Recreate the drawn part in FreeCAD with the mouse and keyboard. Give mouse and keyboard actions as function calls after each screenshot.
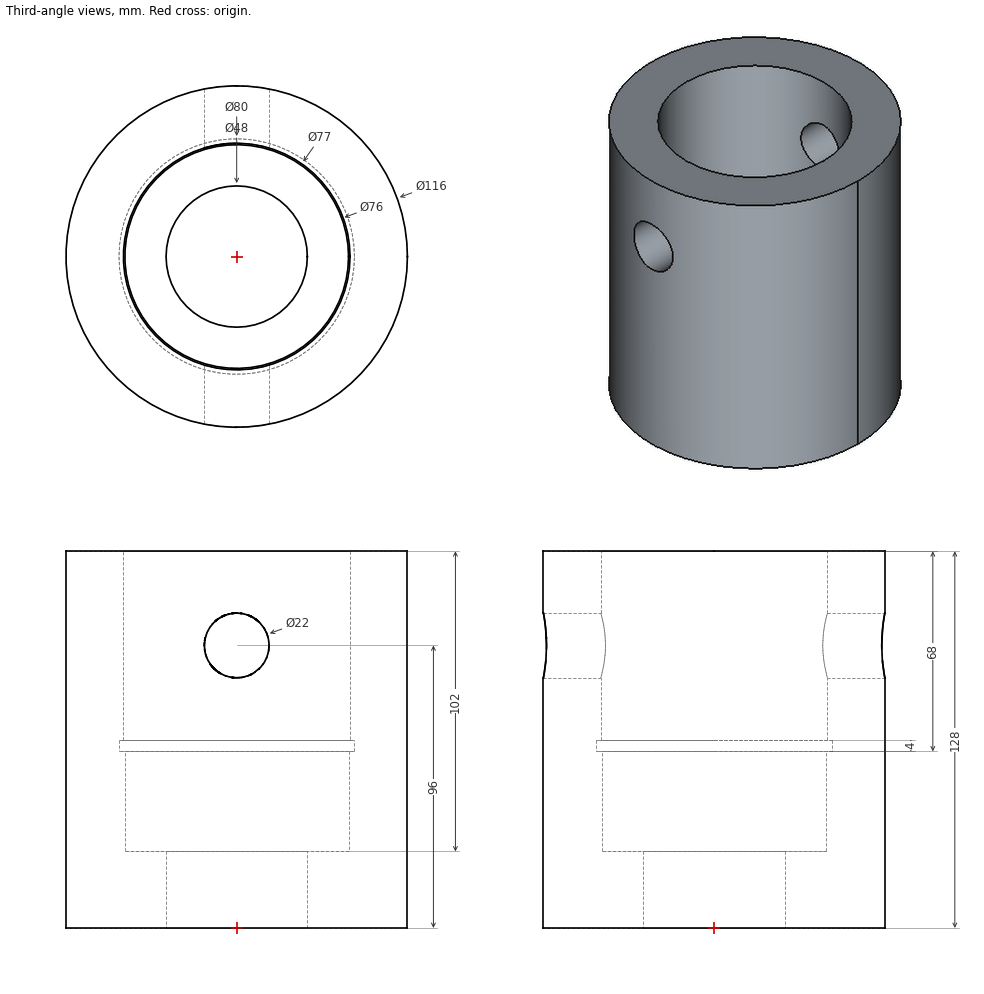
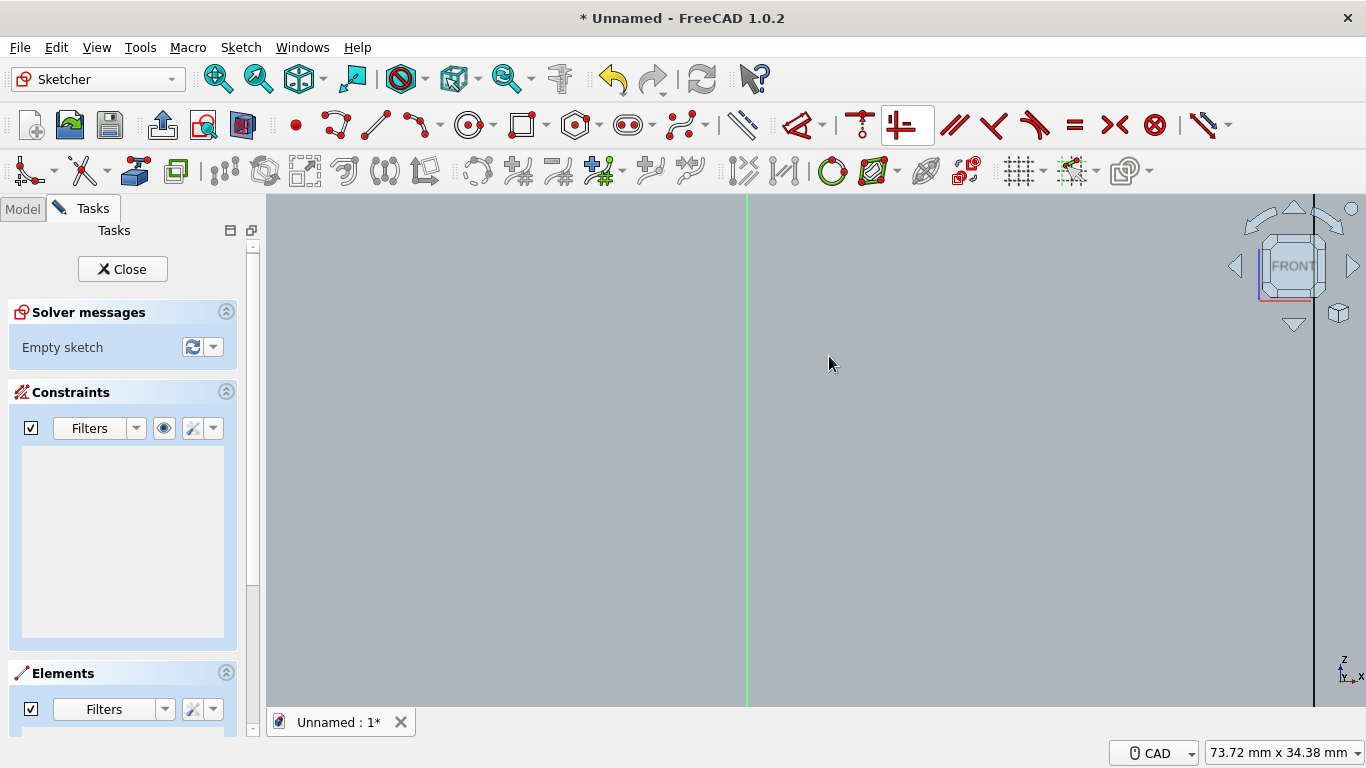
key(g)
key(c)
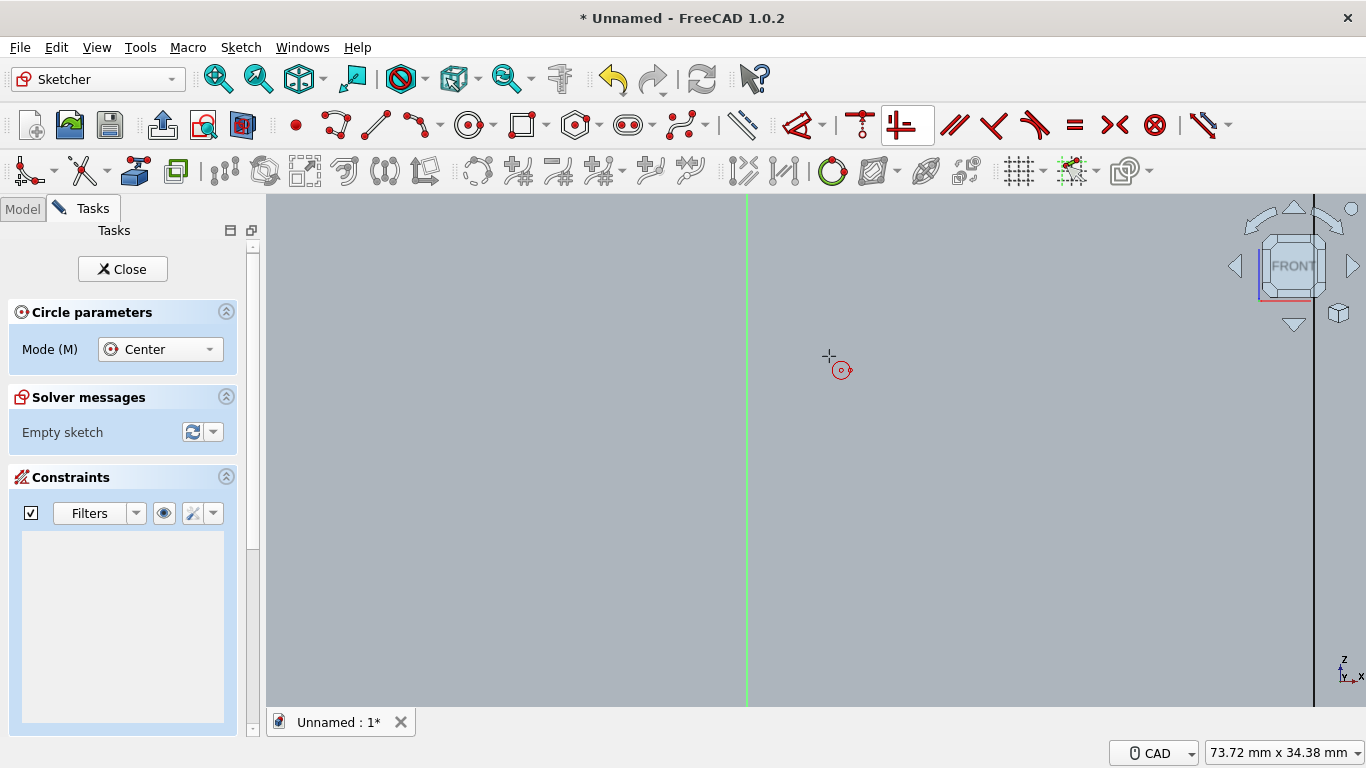
click(747, 449)
move(863, 333)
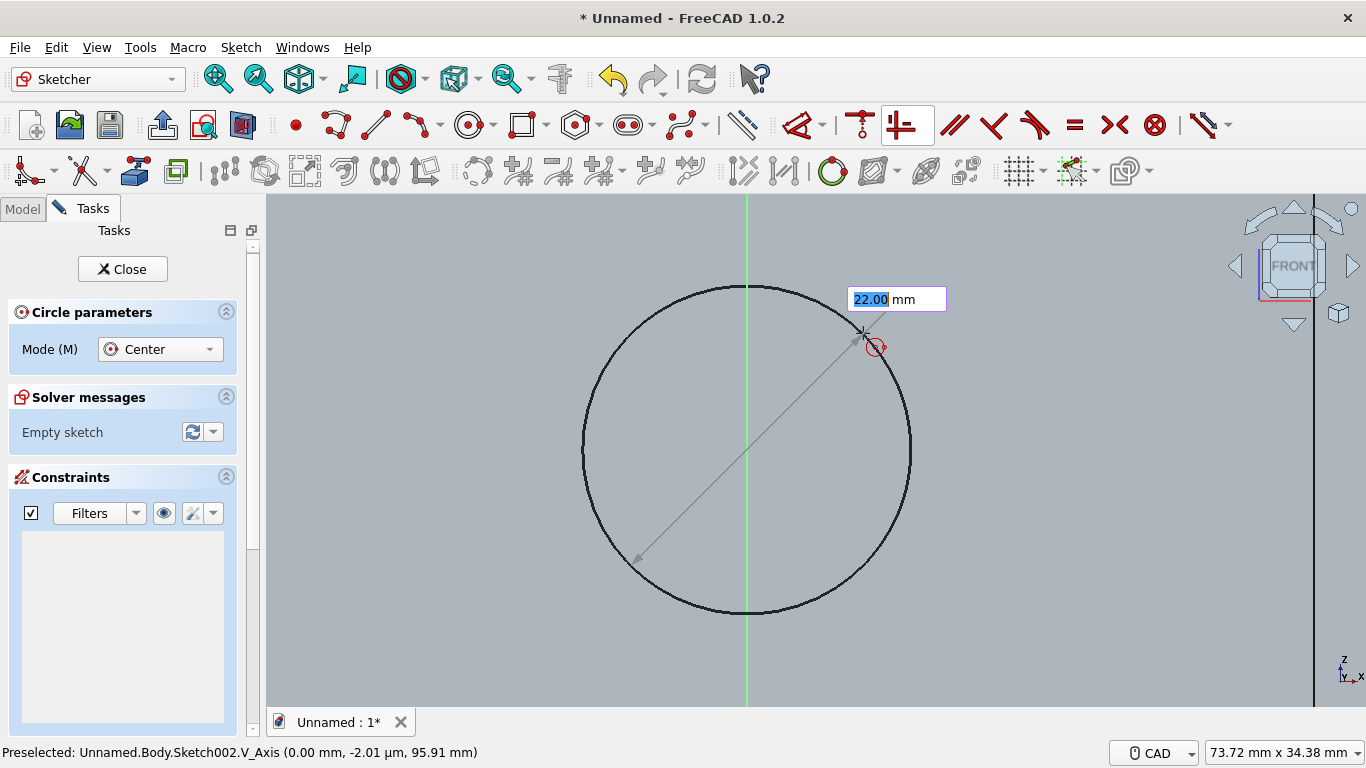
text(22)
key(Return)
key(Escape)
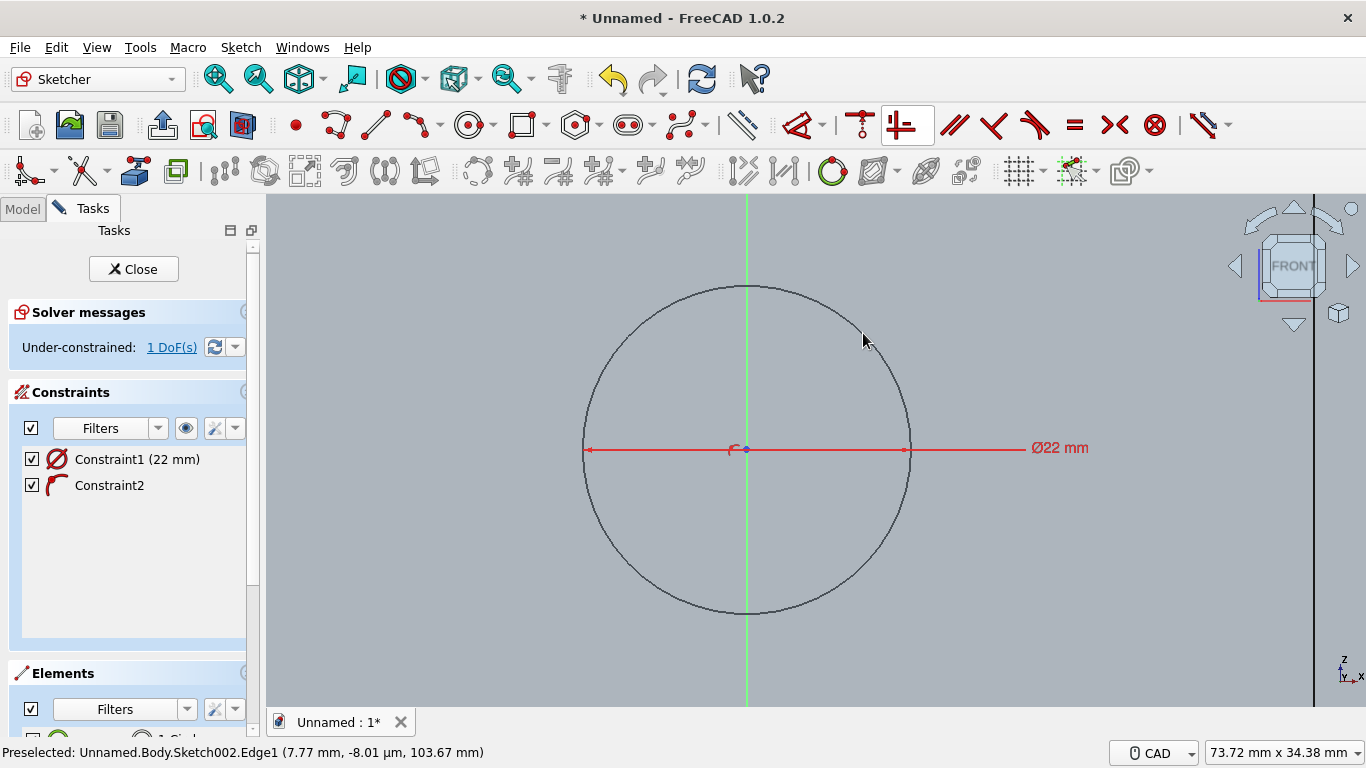
key(d)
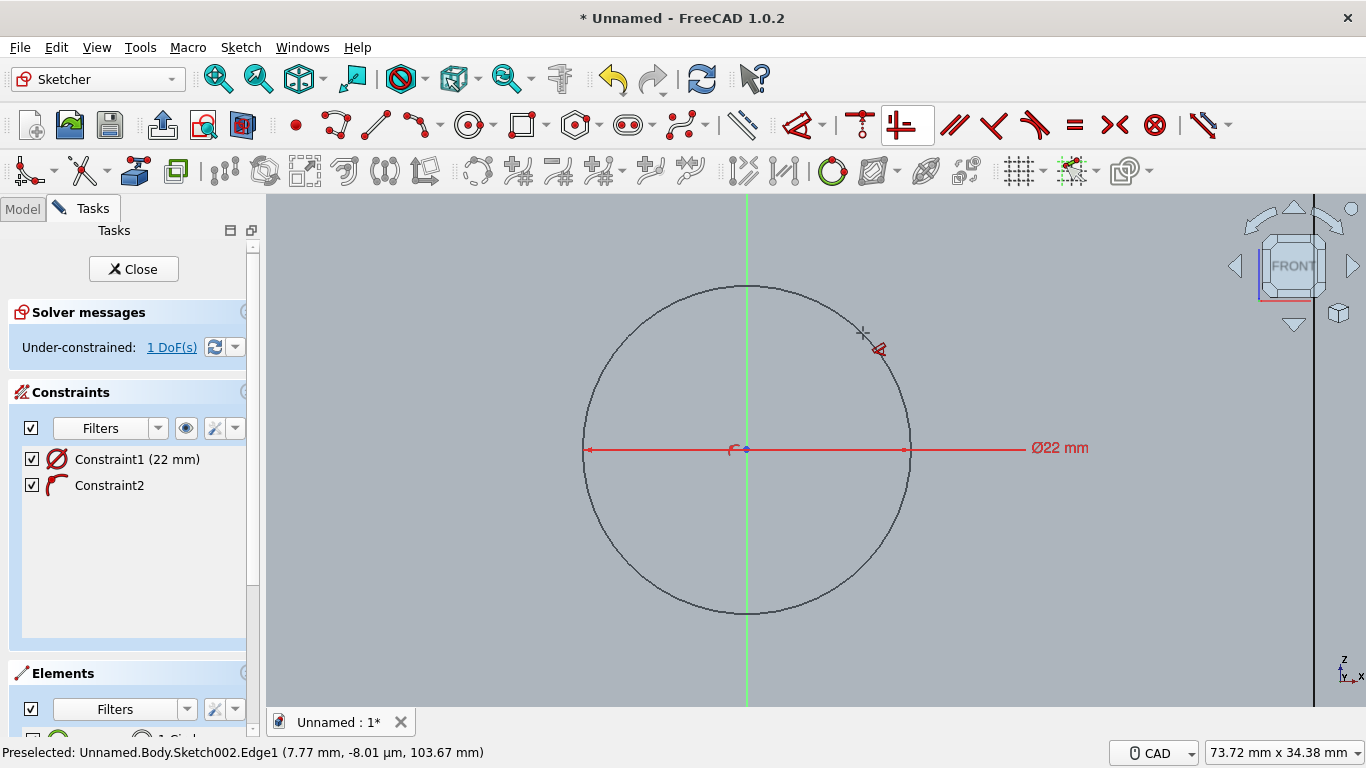
click(747, 450)
click(781, 564)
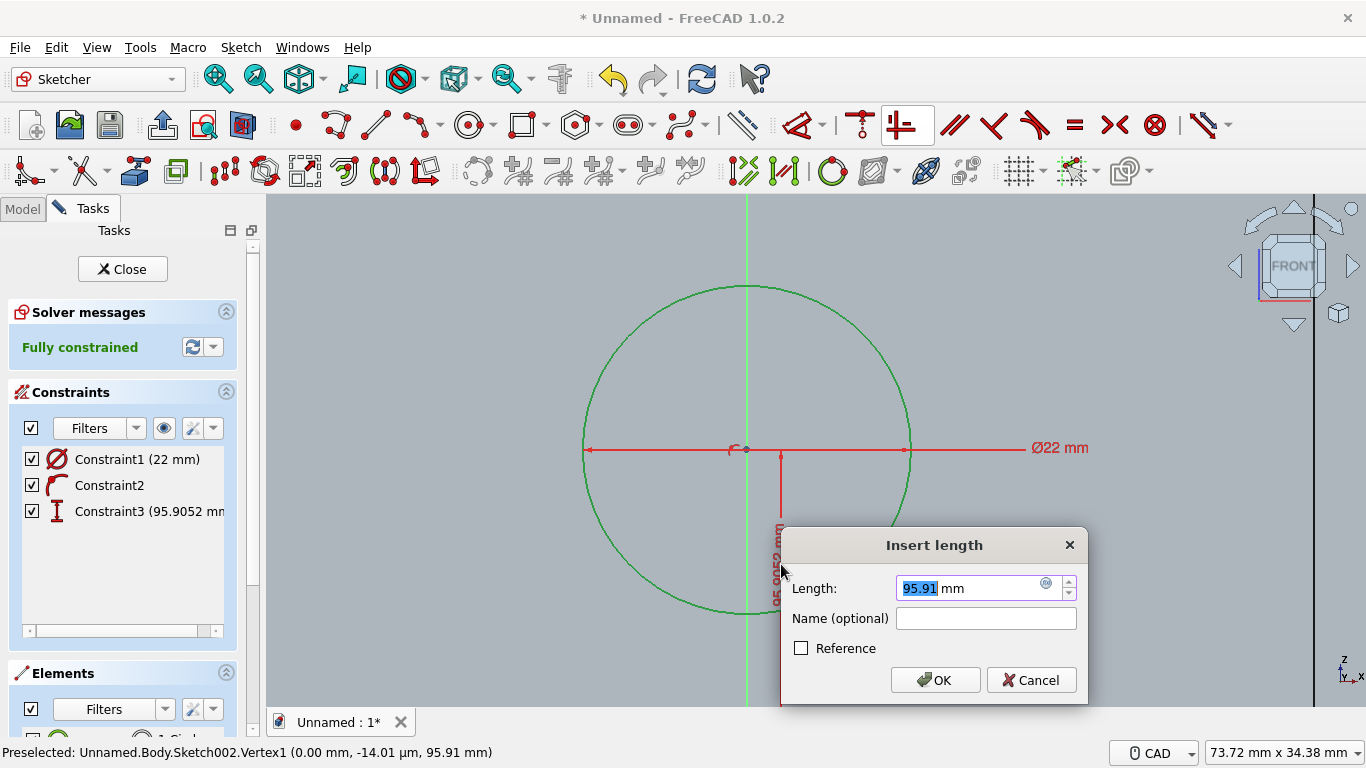
text(96)
key(Return)
key(Escape)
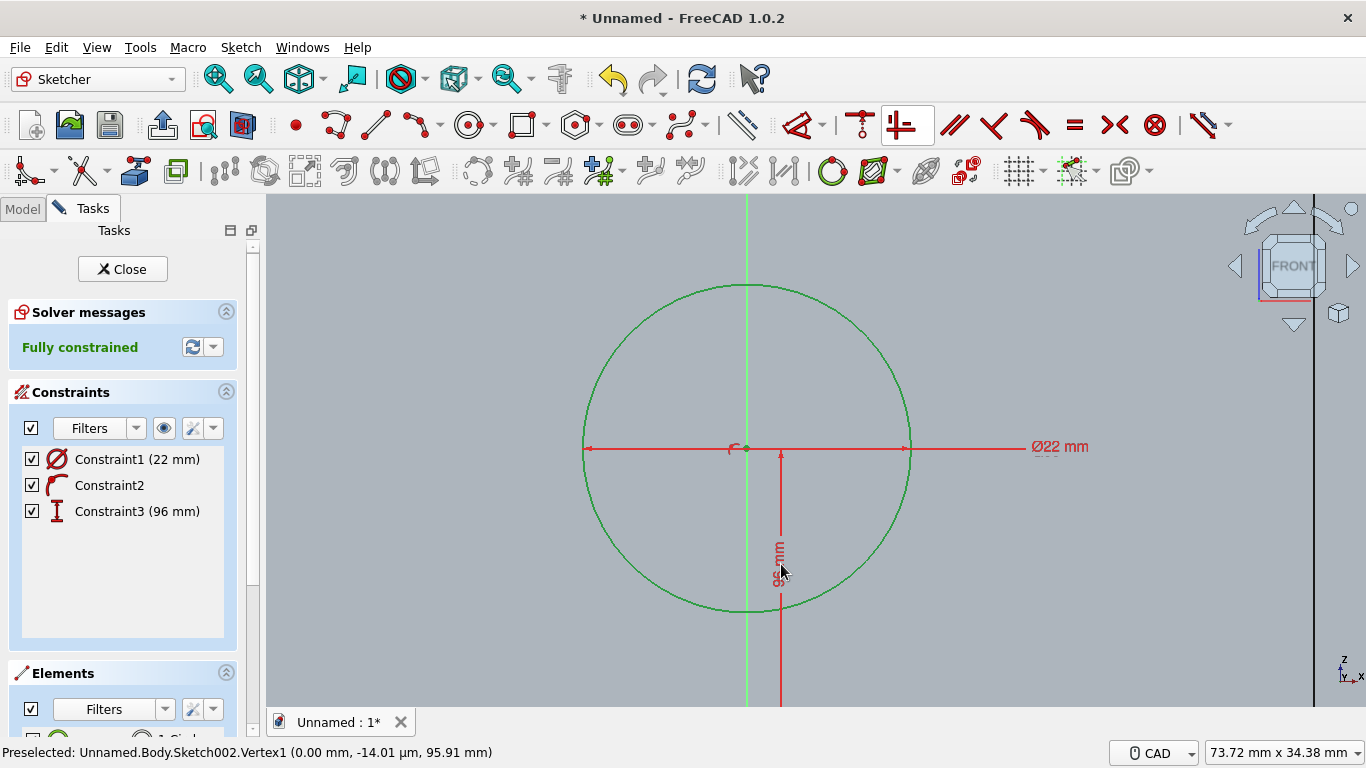
click(123, 269)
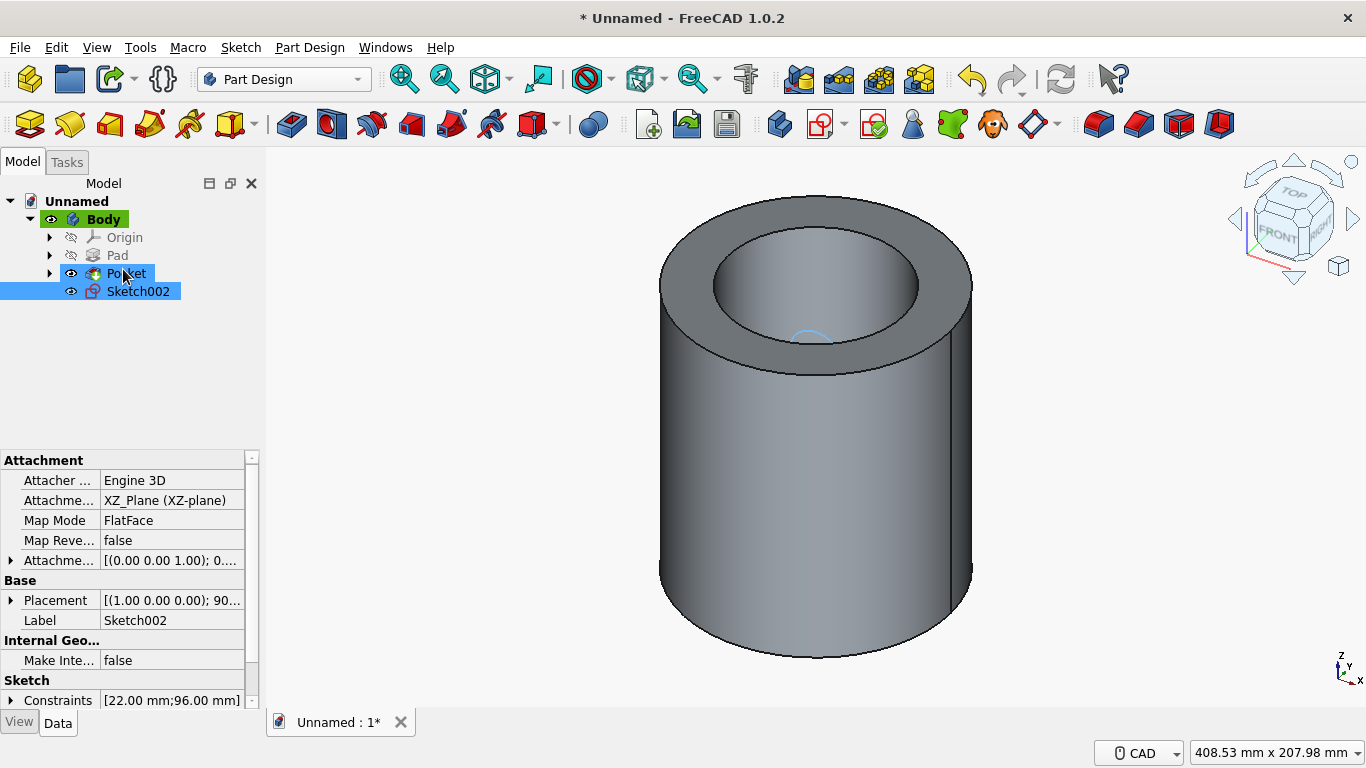
click(292, 124)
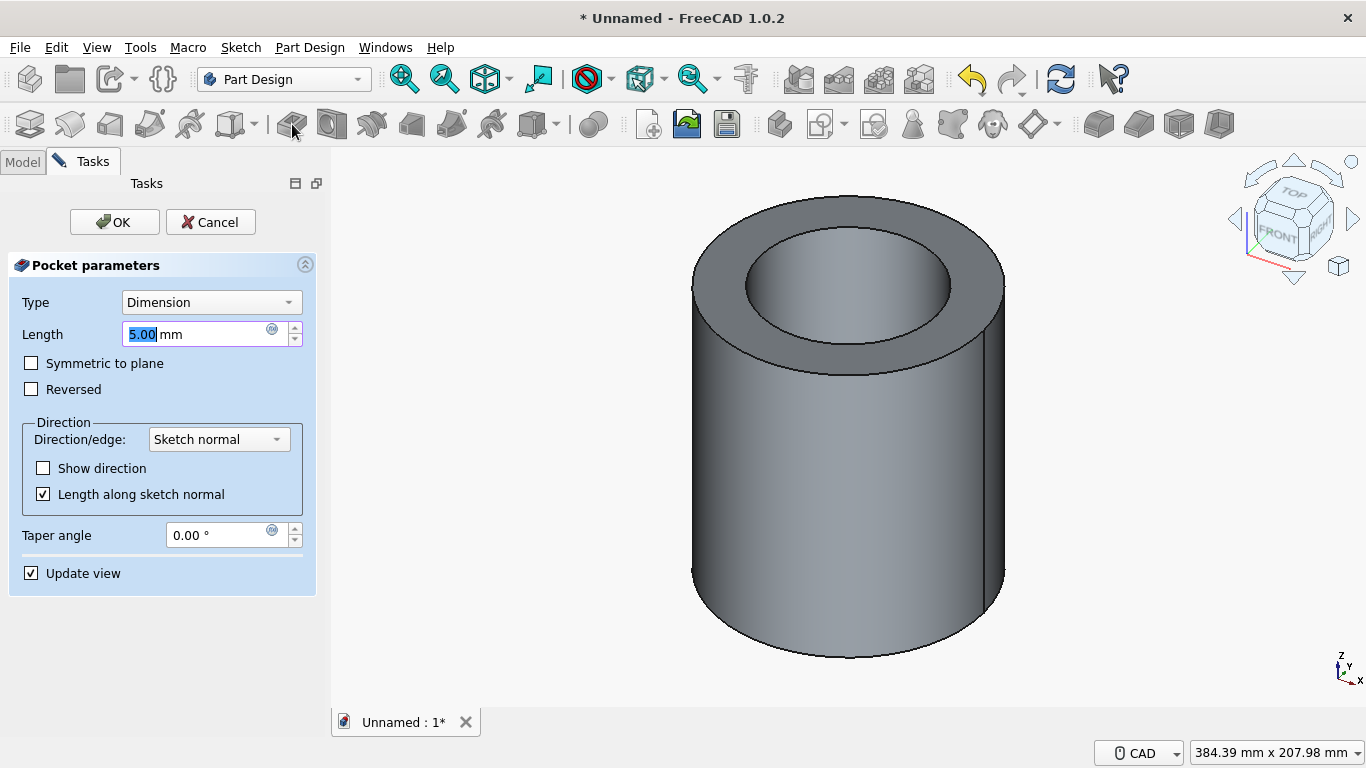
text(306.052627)
key(Tab)